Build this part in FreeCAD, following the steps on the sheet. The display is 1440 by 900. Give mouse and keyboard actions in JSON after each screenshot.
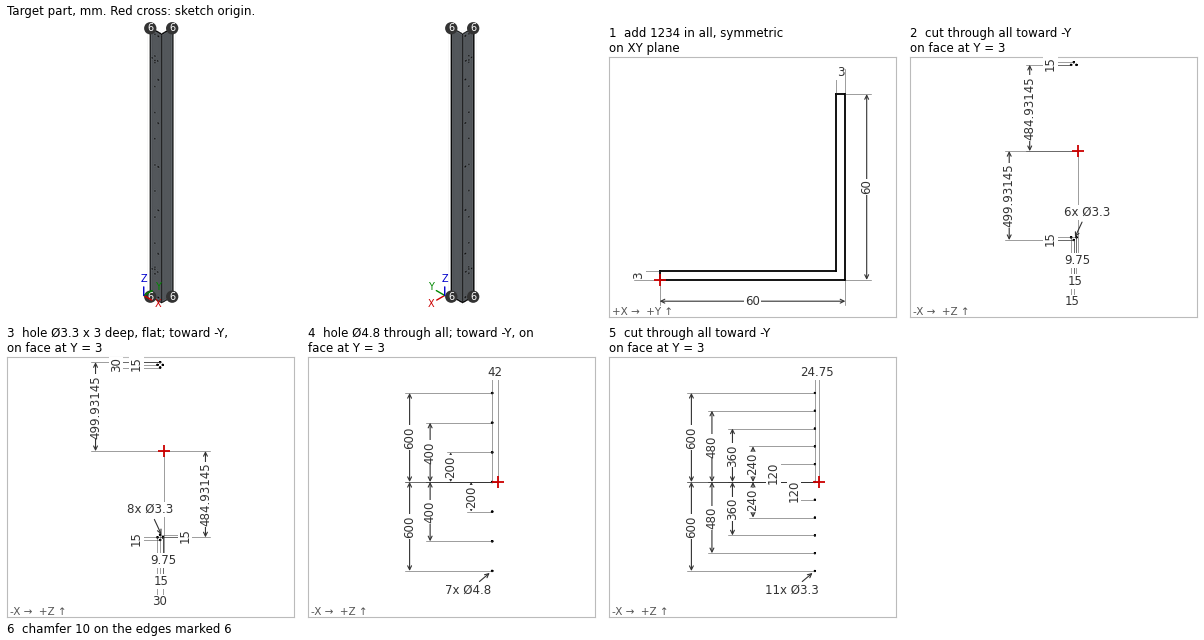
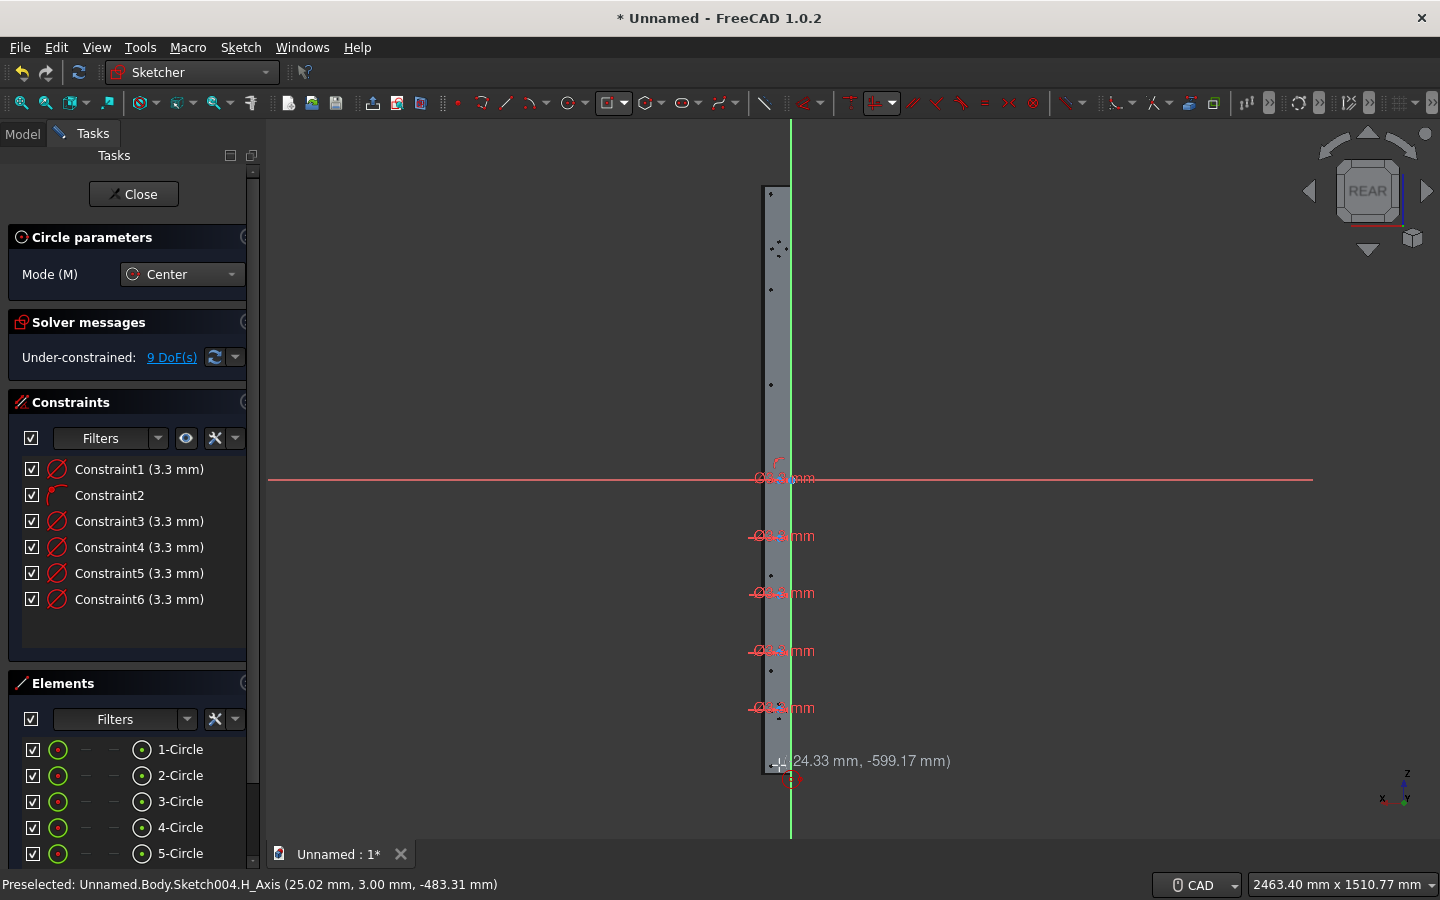
{"action": "scroll", "coordinate": [779, 766], "scroll_direction": "up", "scroll_amount": 2}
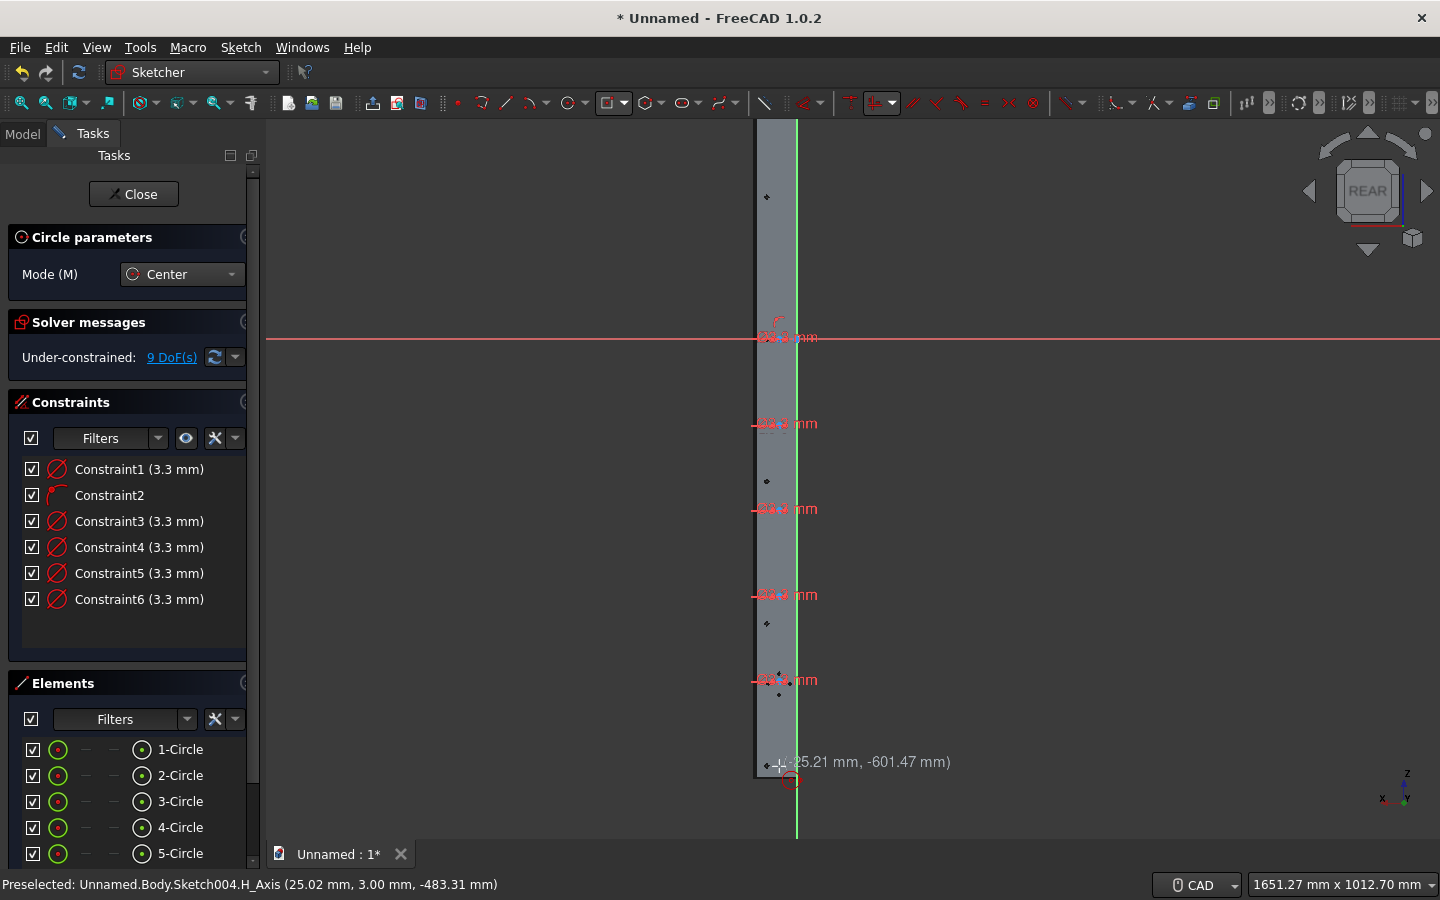
{"action": "left_click", "coordinate": [779, 766]}
{"action": "mouse_move", "coordinate": [780, 765]}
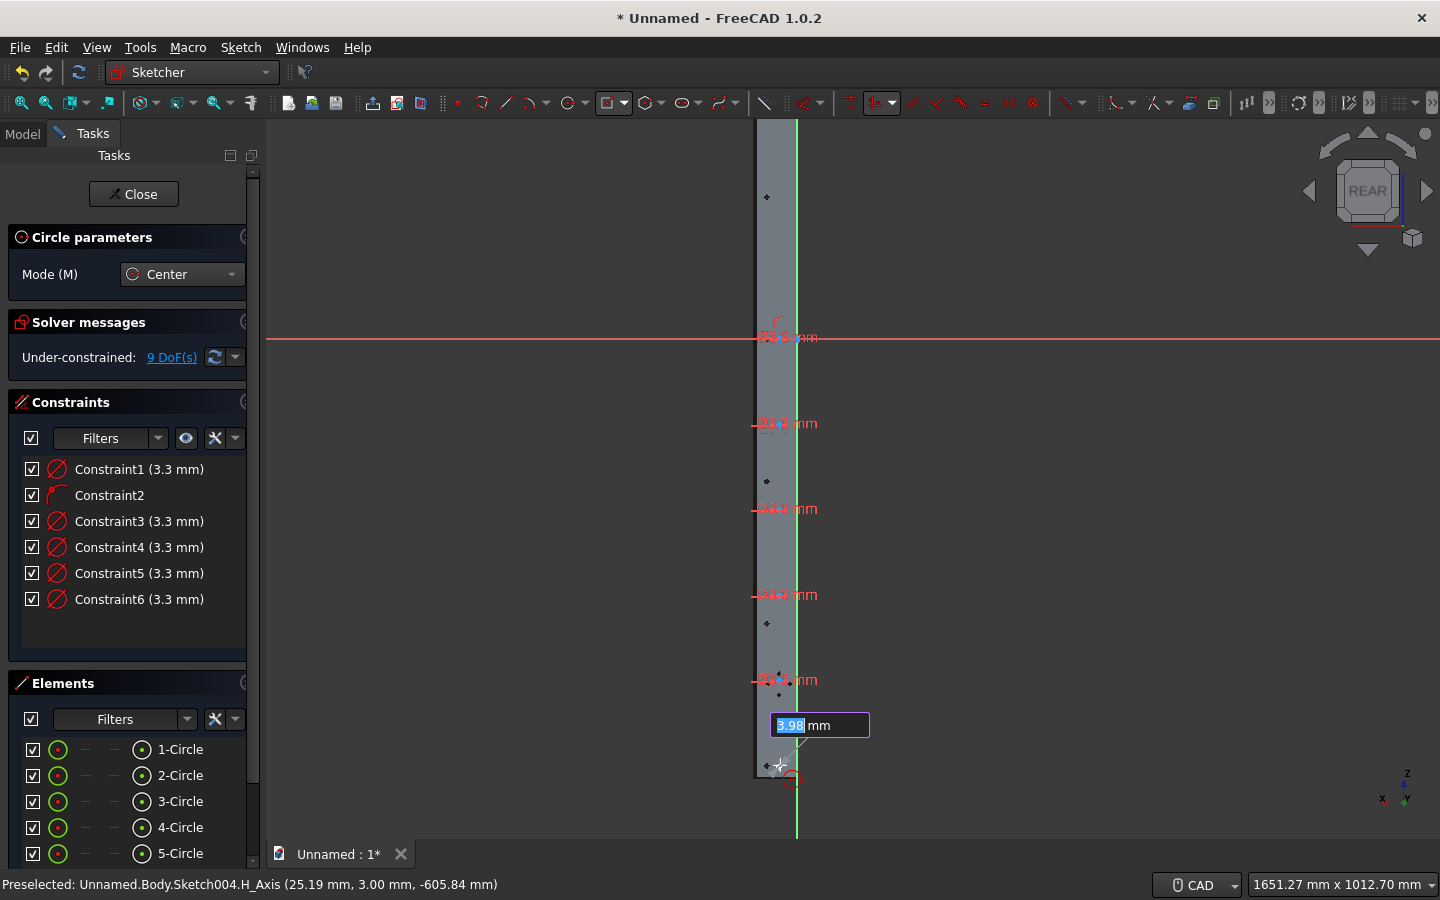
{"action": "type", "text": "3.3"}
{"action": "key", "text": "Return"}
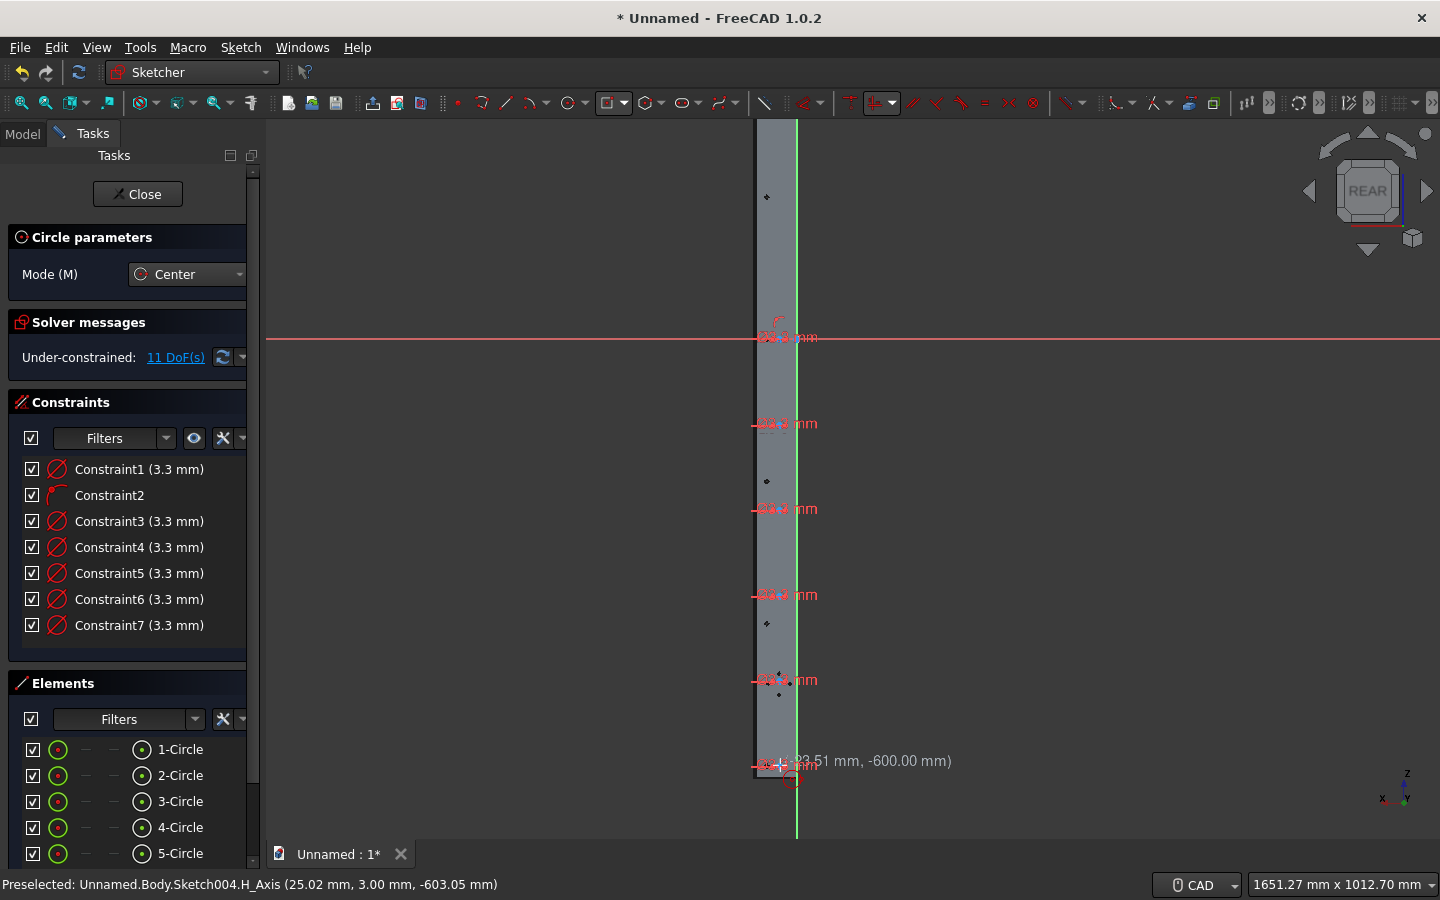
{"action": "scroll", "coordinate": [781, 649], "scroll_direction": "down", "scroll_amount": 3}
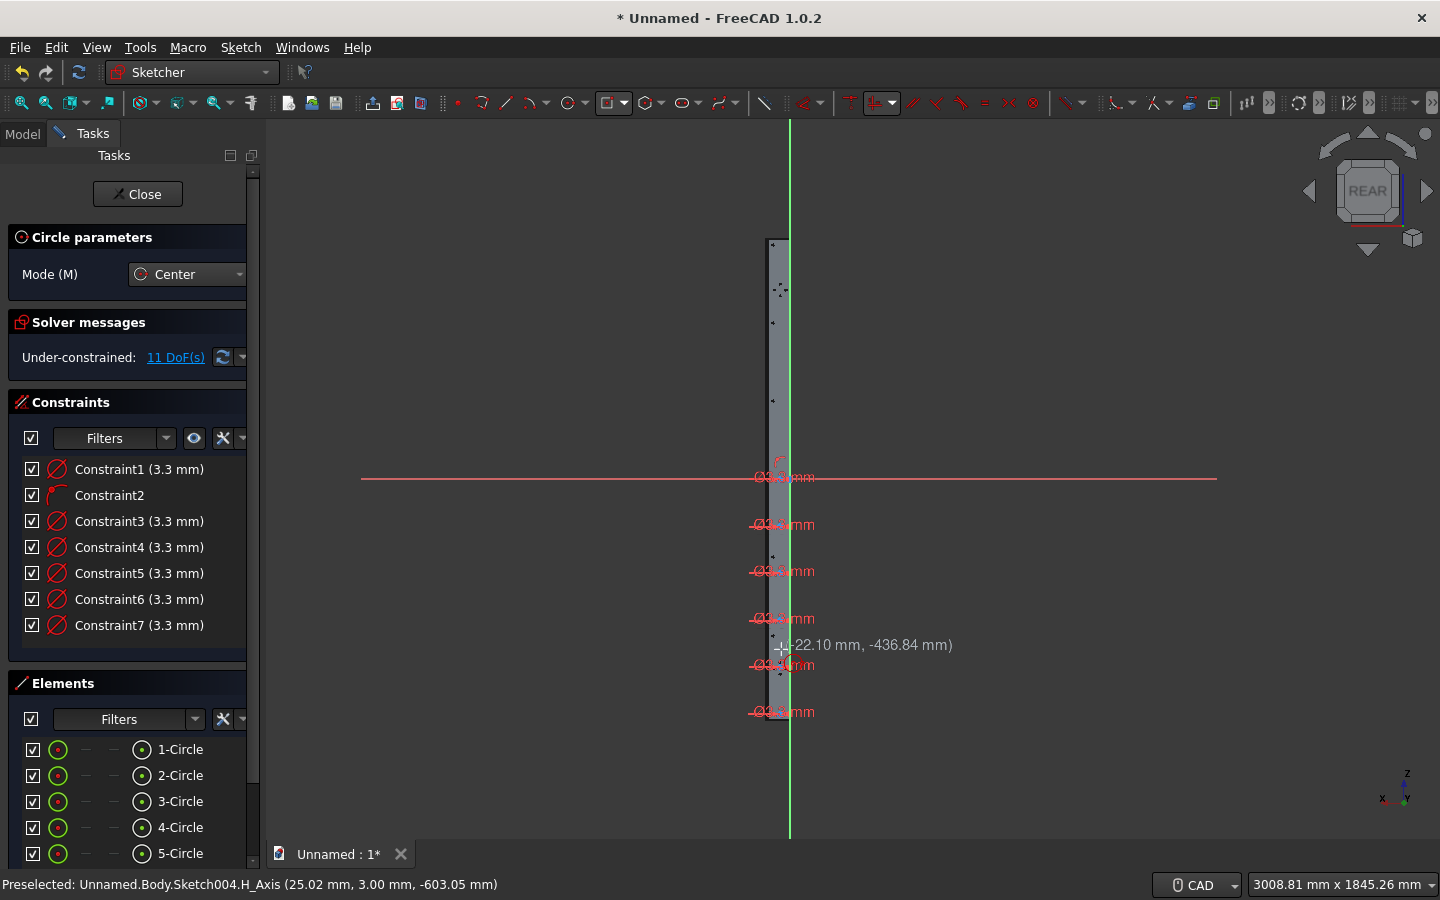
{"action": "scroll", "coordinate": [780, 245], "scroll_direction": "up", "scroll_amount": 18}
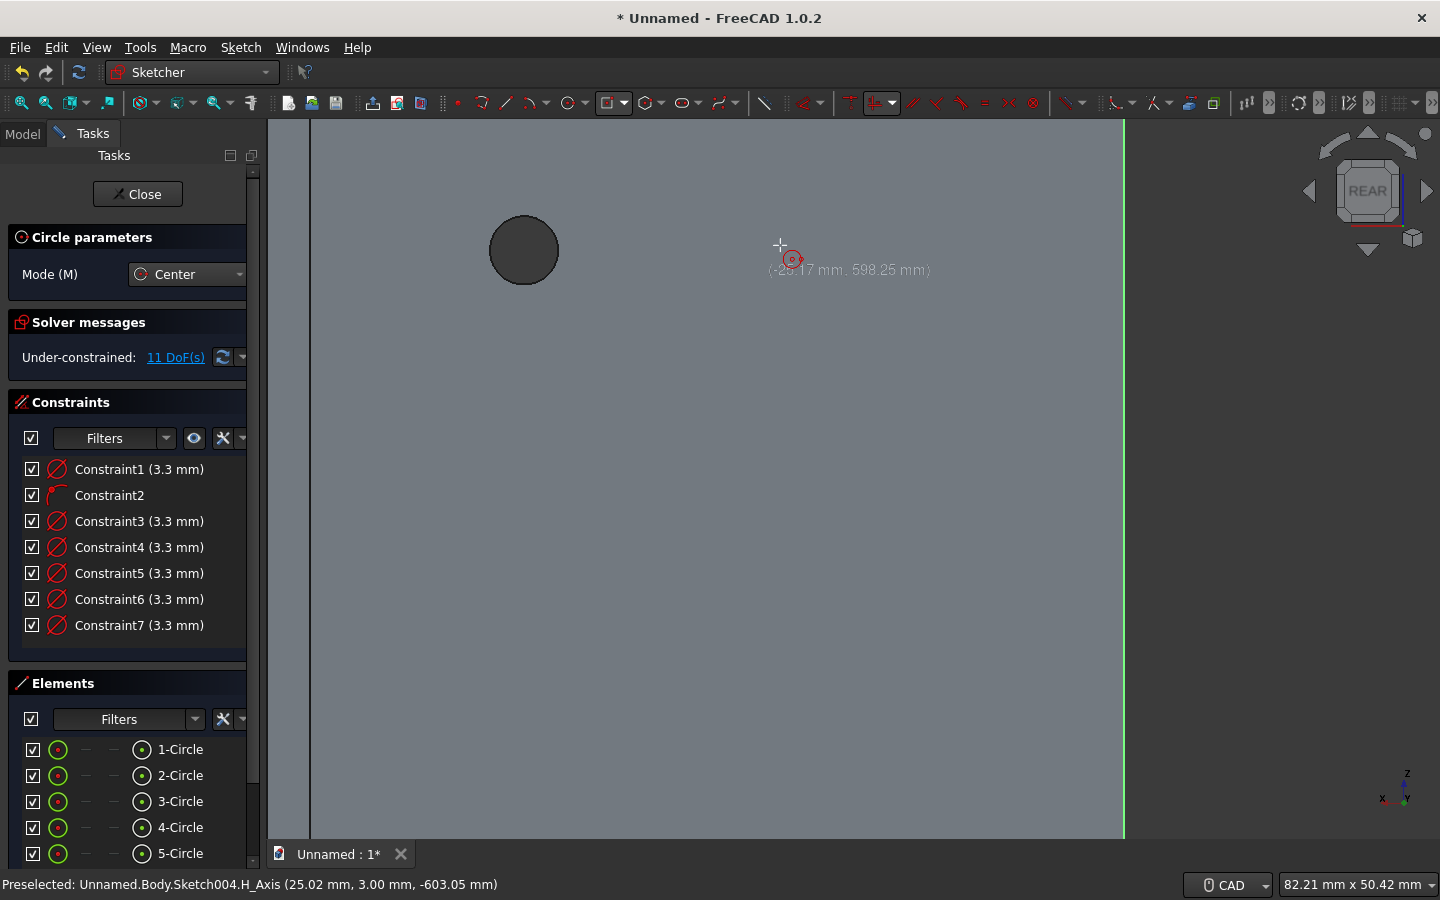
{"action": "scroll", "coordinate": [779, 191], "scroll_direction": "down", "scroll_amount": 17}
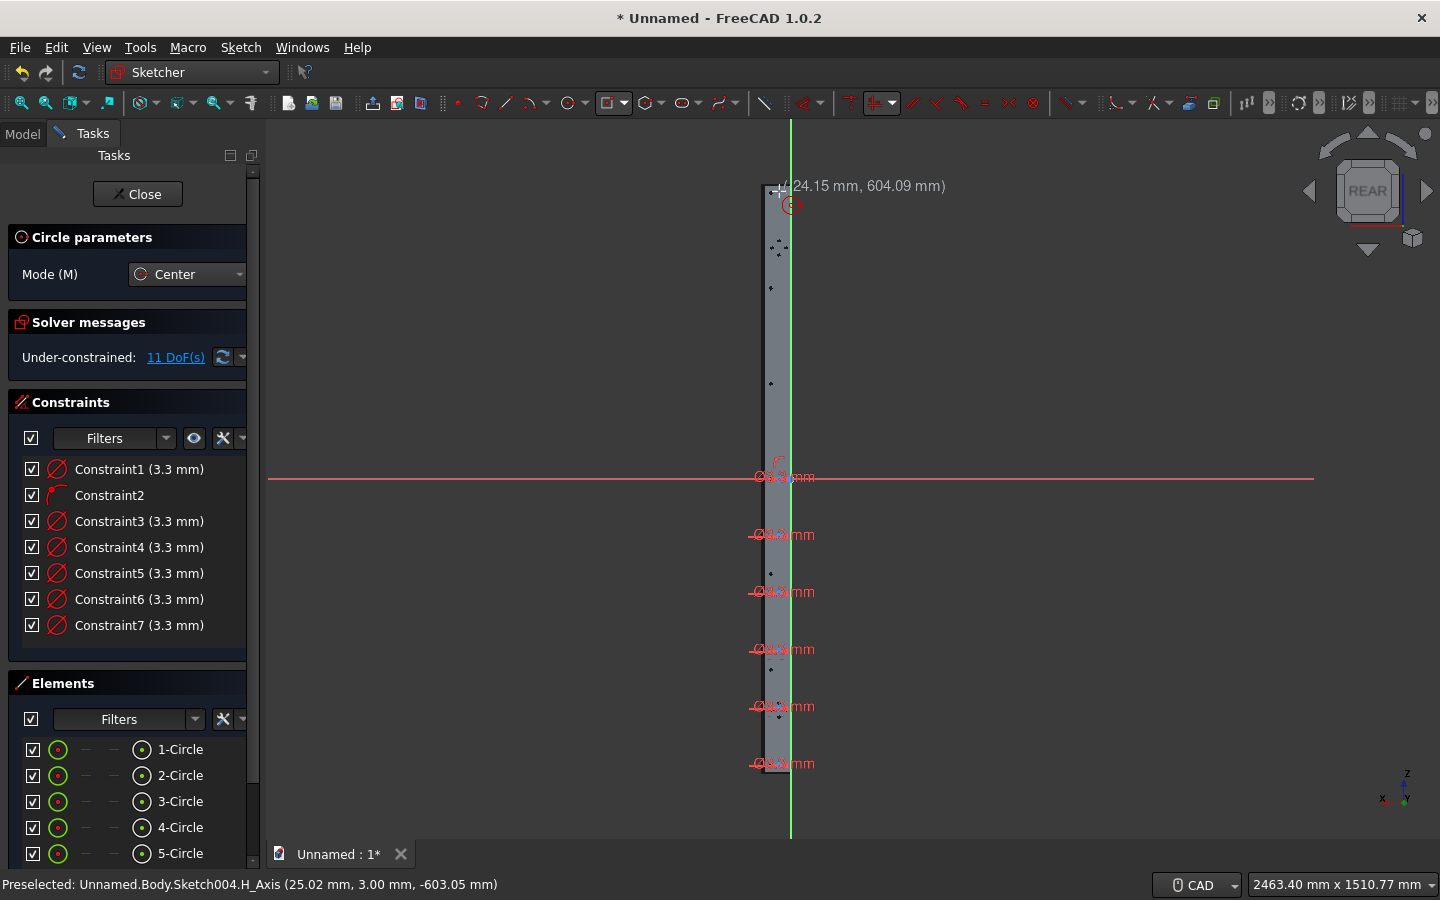
{"action": "scroll", "coordinate": [779, 193], "scroll_direction": "up", "scroll_amount": 2}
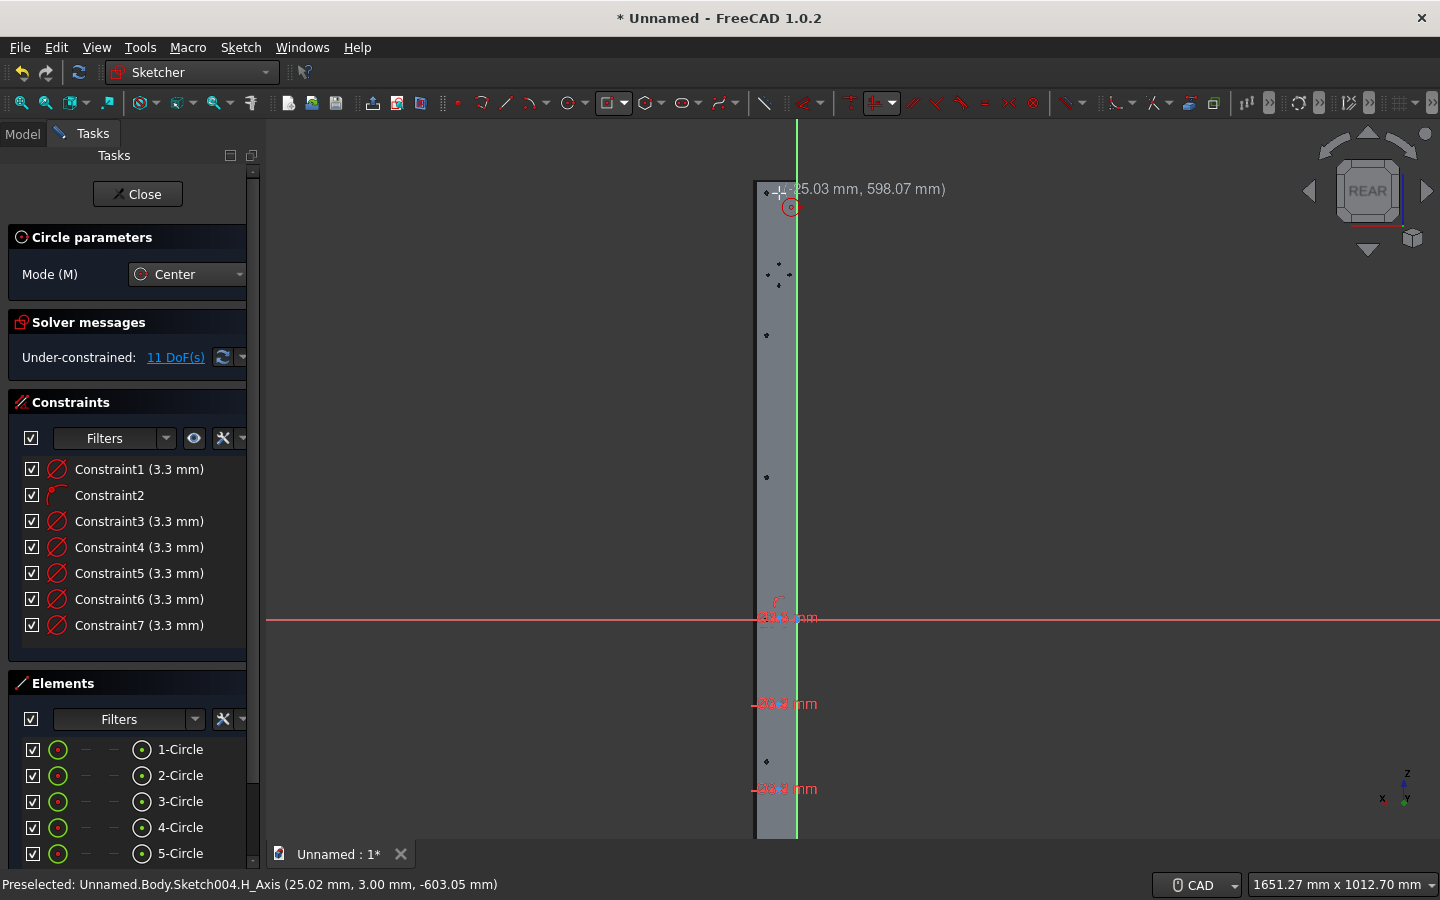
{"action": "left_click", "coordinate": [779, 193]}
{"action": "mouse_move", "coordinate": [780, 192]}